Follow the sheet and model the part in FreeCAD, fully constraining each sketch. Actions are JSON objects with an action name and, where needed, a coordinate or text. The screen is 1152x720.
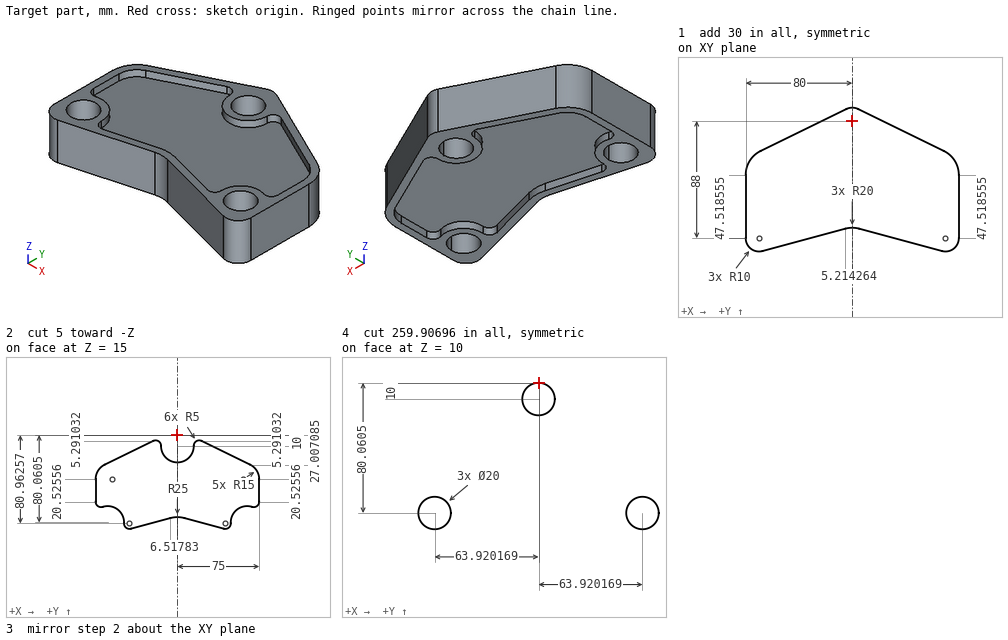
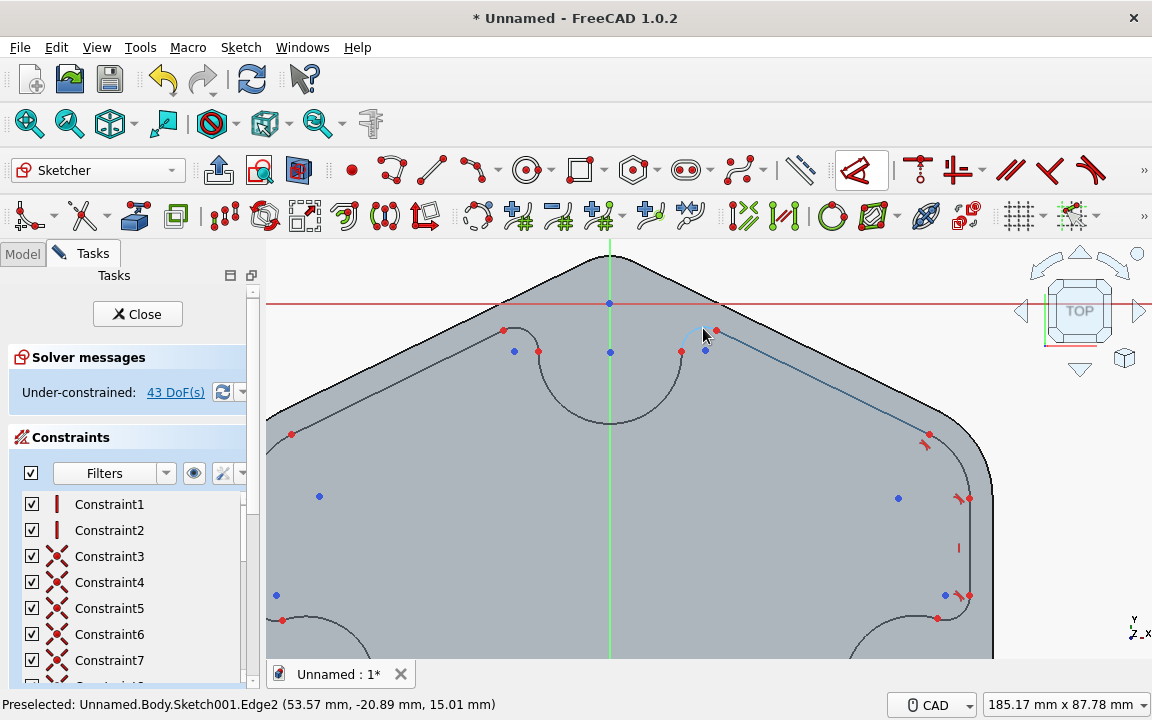
{"action": "left_click", "coordinate": [702, 328]}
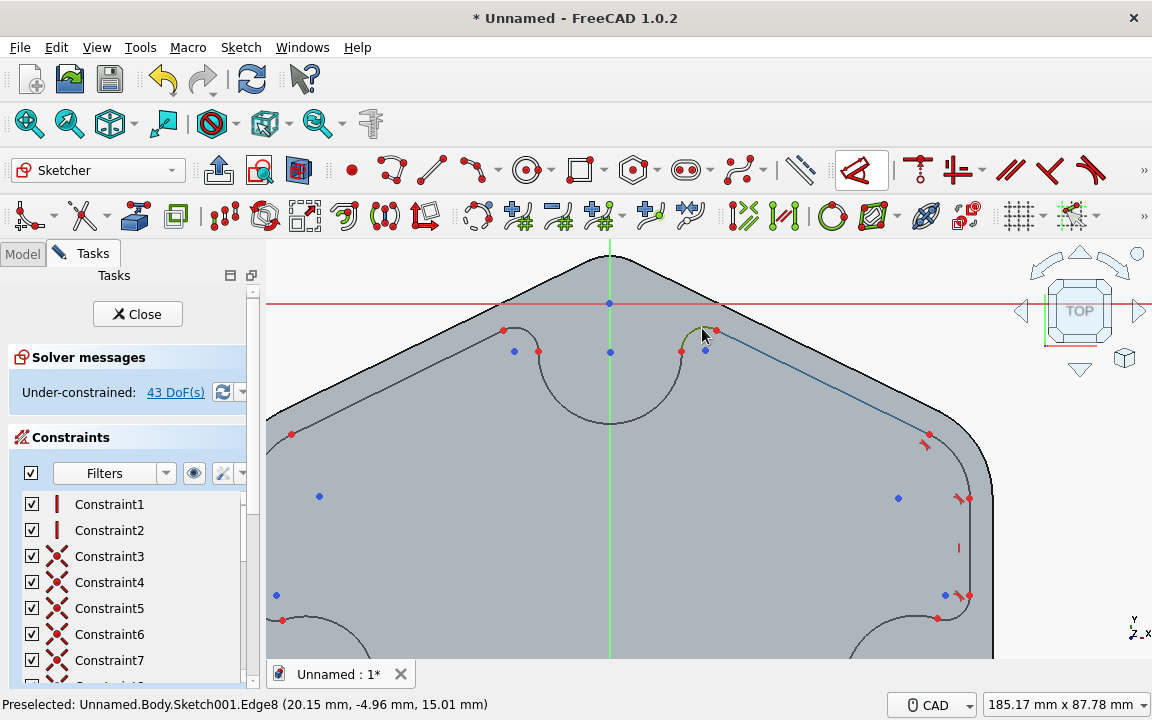
{"action": "key", "text": "t"}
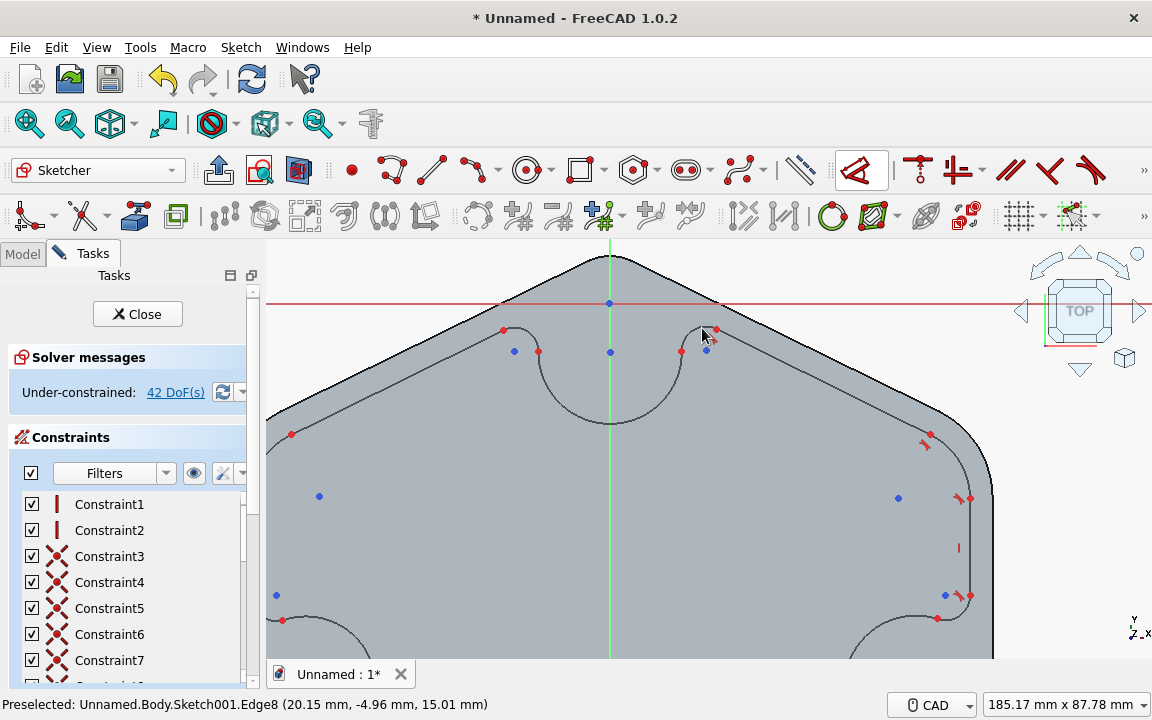
{"action": "left_click", "coordinate": [440, 362]}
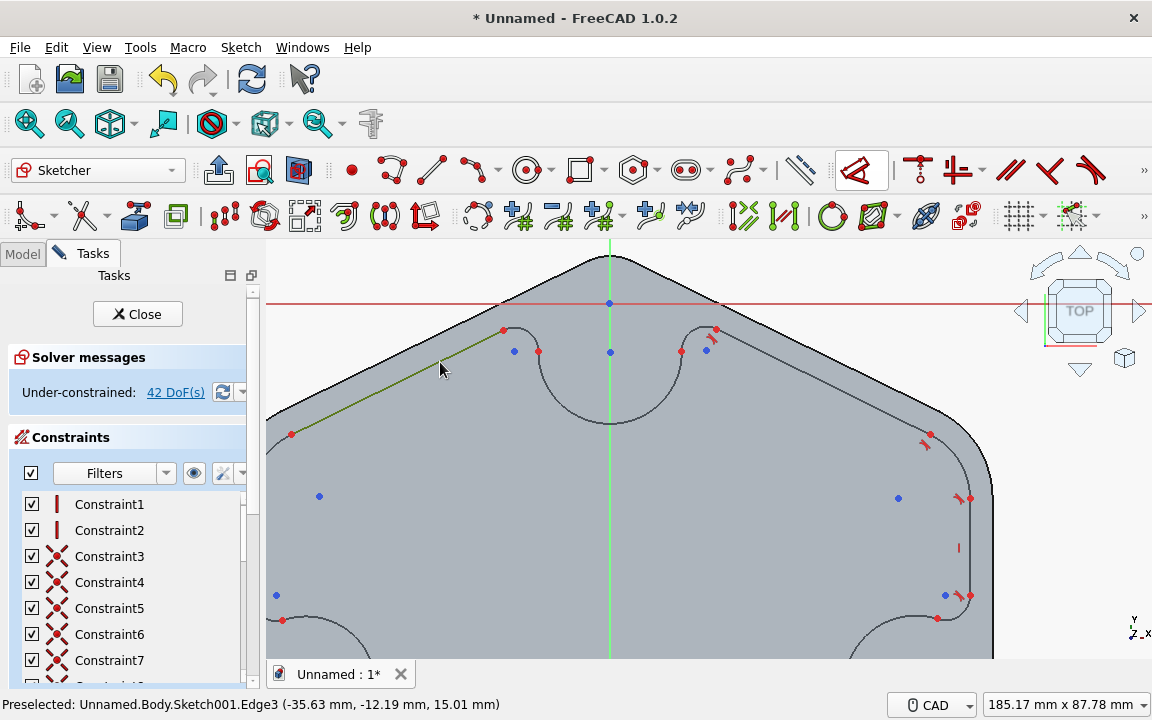
{"action": "left_click", "coordinate": [534, 337]}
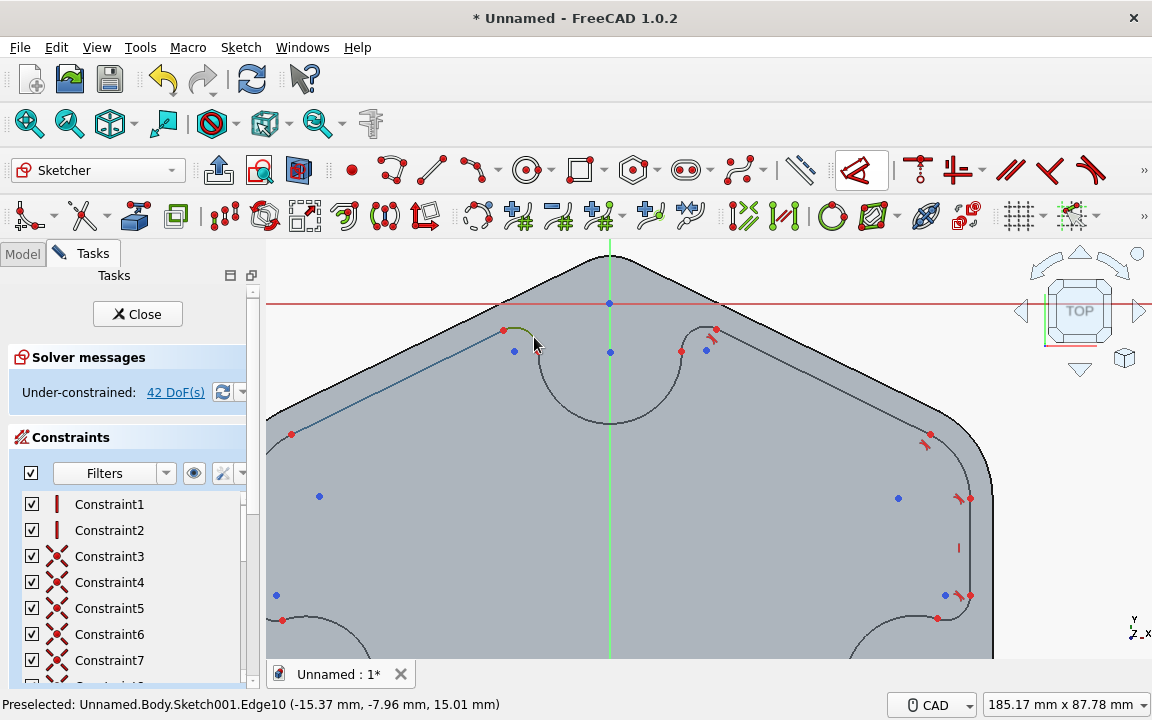
{"action": "left_click", "coordinate": [1092, 170]}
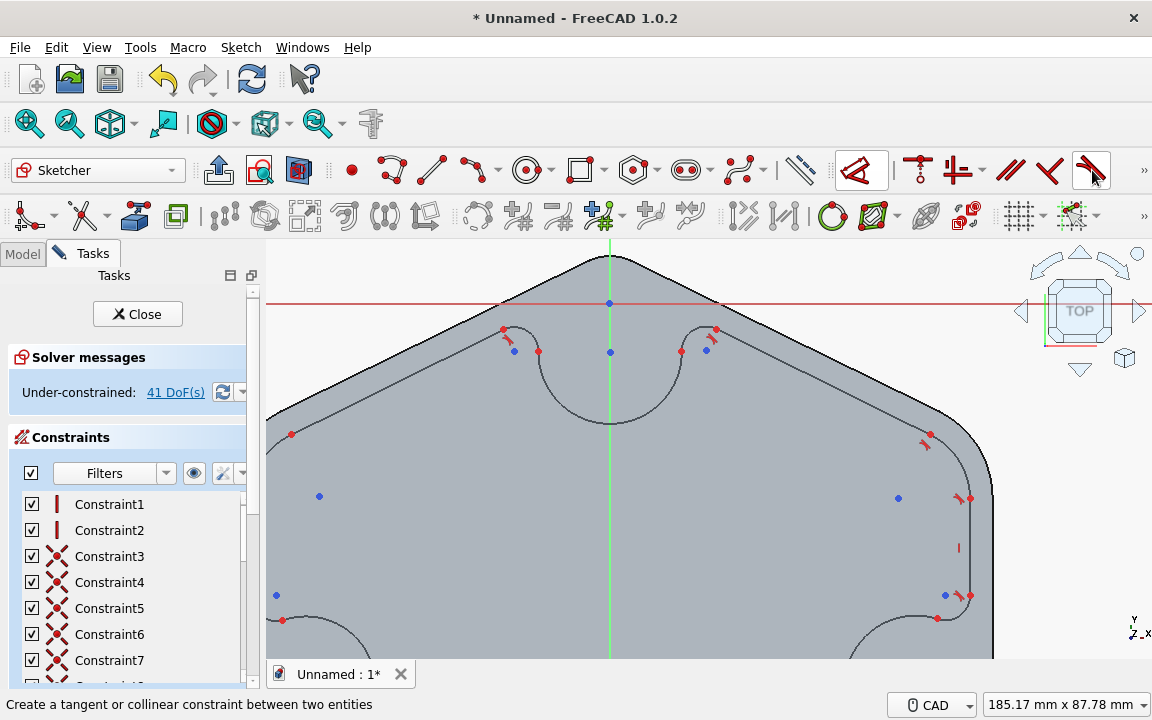
{"action": "left_click", "coordinate": [440, 361]}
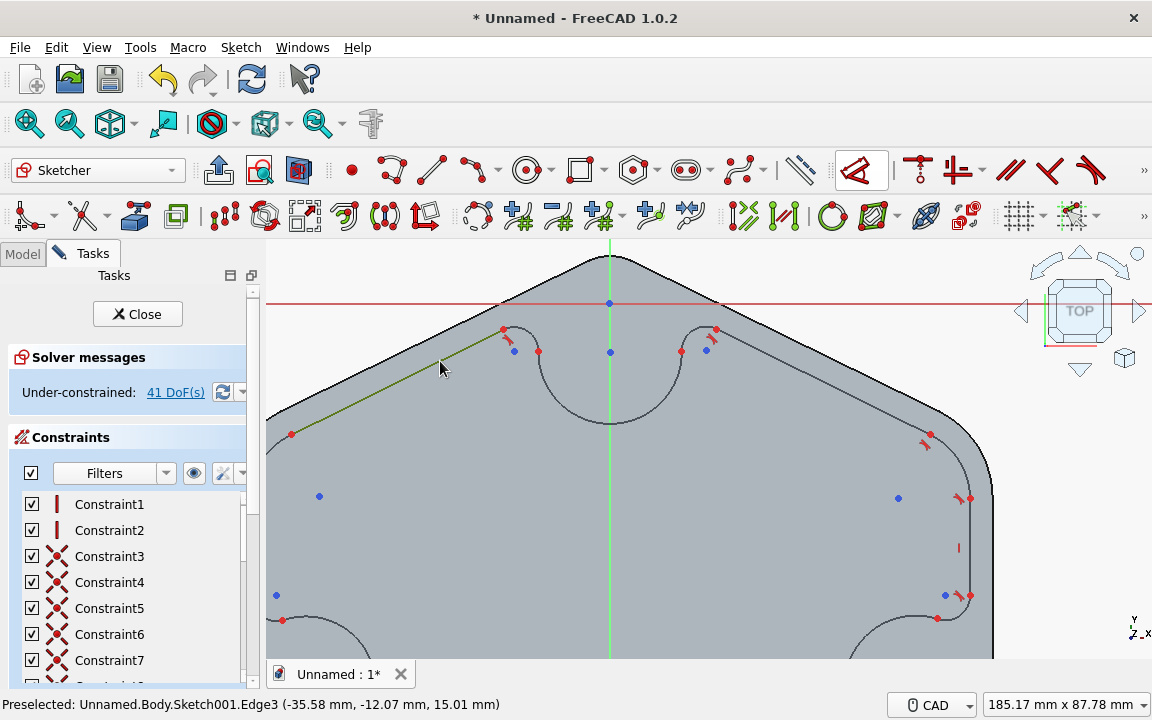
{"action": "scroll", "coordinate": [703, 327], "scroll_direction": "down", "scroll_amount": 2}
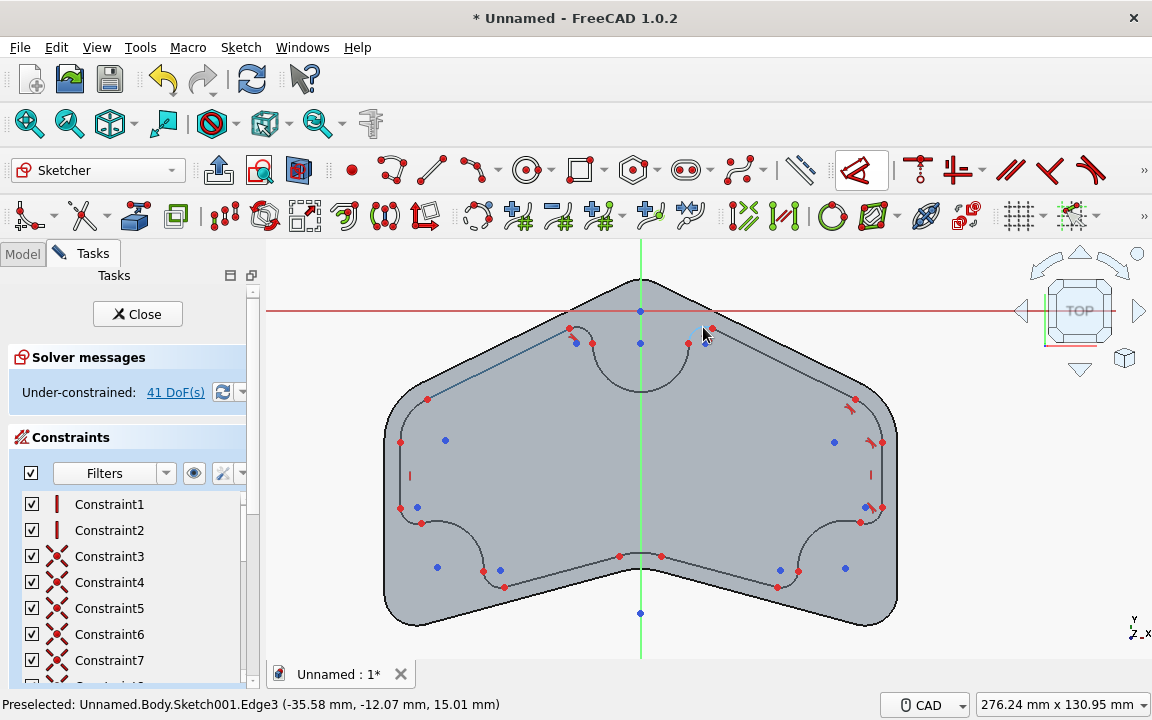
{"action": "left_click", "coordinate": [414, 408]}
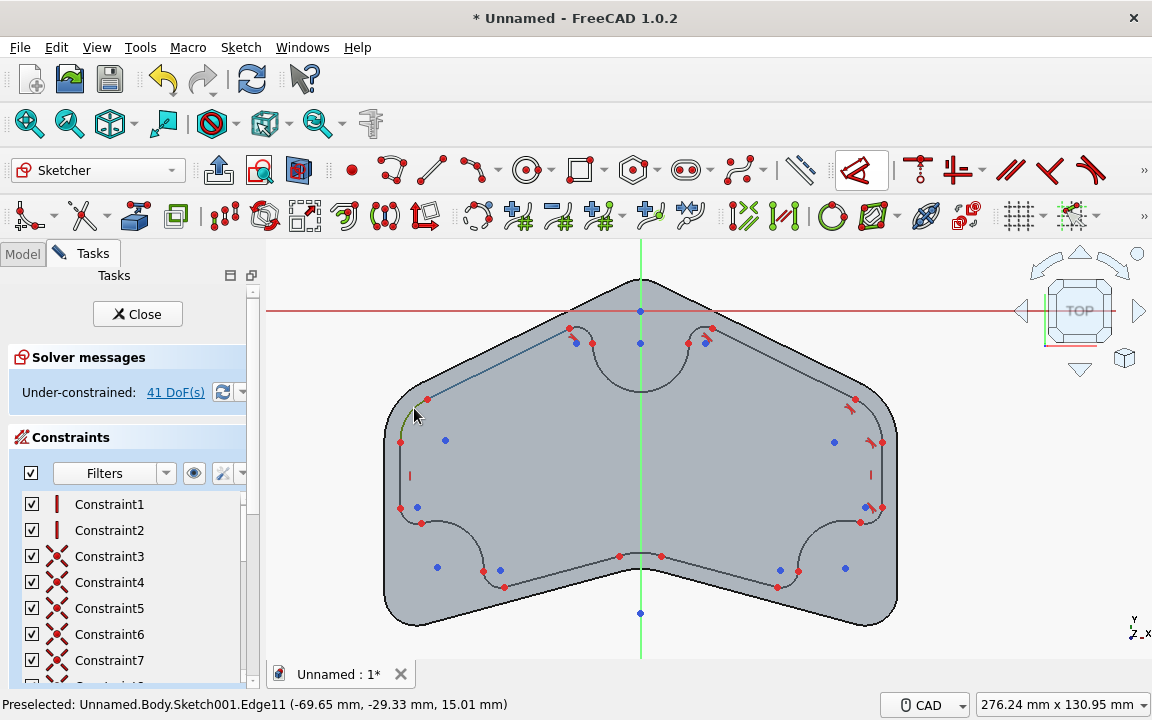
{"action": "key", "text": "t"}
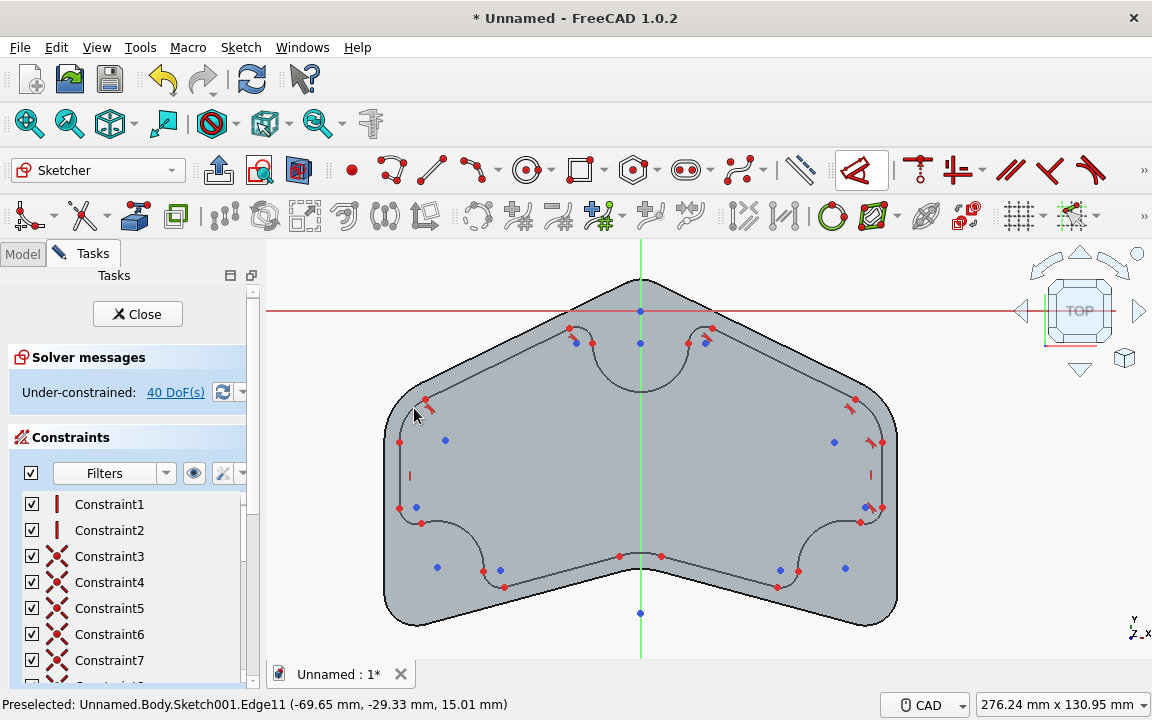
{"action": "left_click", "coordinate": [400, 462]}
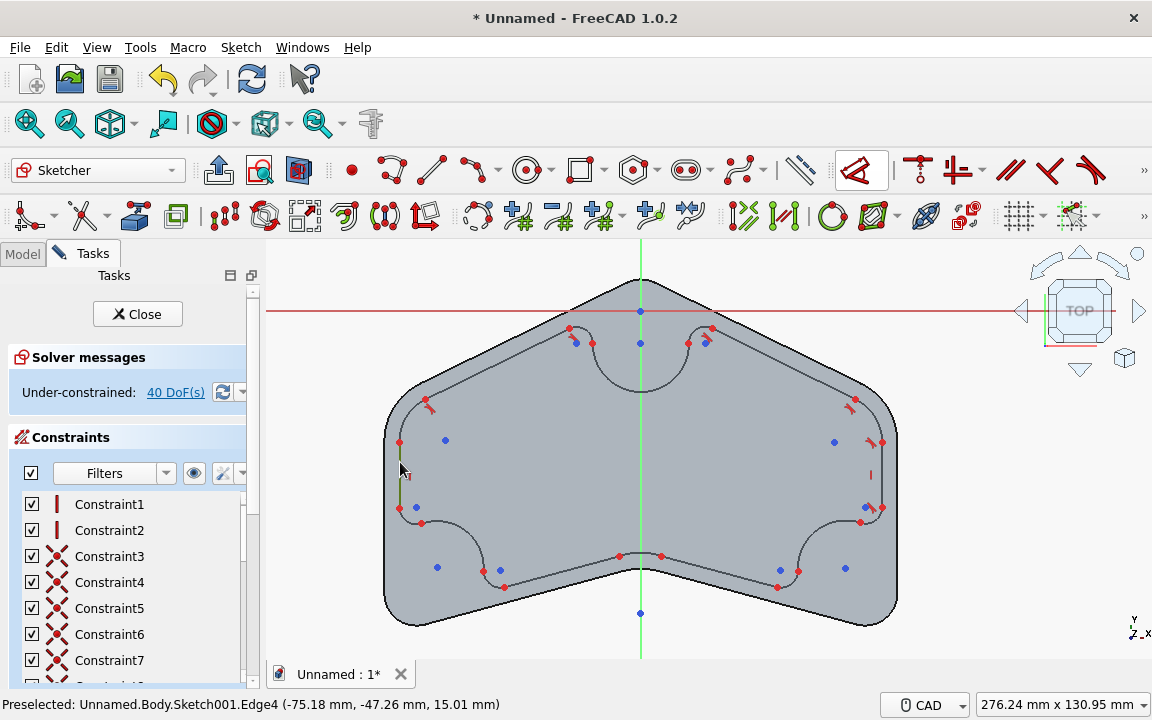
{"action": "left_click", "coordinate": [413, 409]}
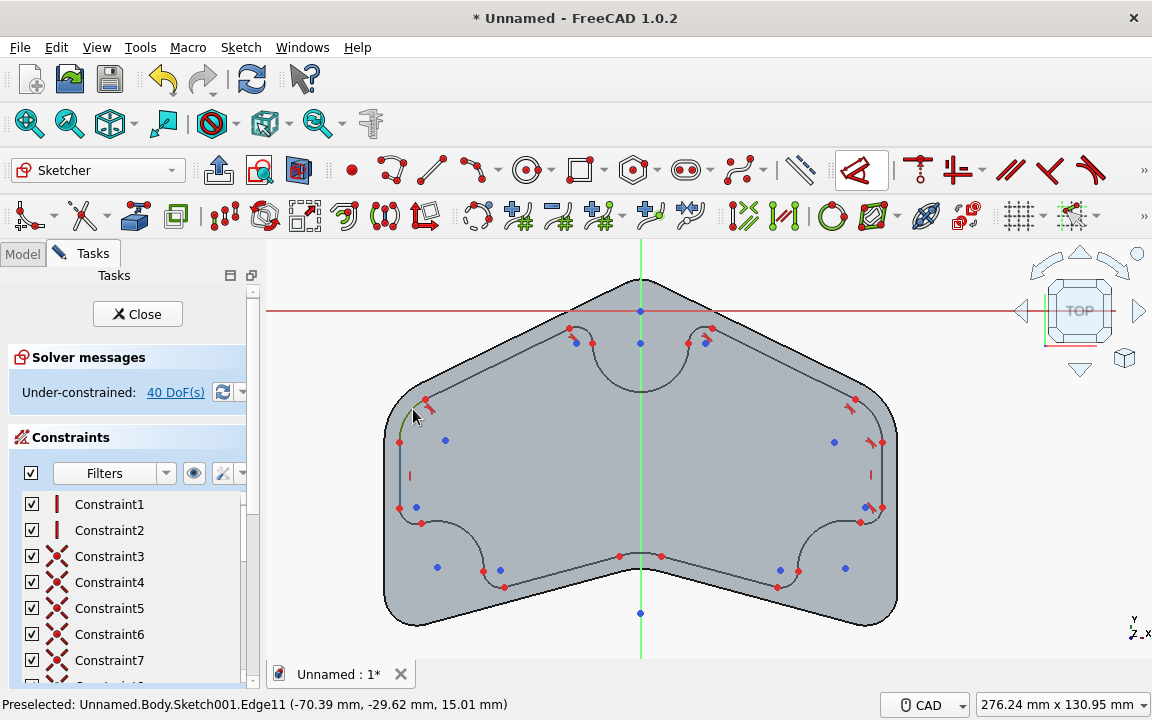
{"action": "left_click", "coordinate": [1092, 170]}